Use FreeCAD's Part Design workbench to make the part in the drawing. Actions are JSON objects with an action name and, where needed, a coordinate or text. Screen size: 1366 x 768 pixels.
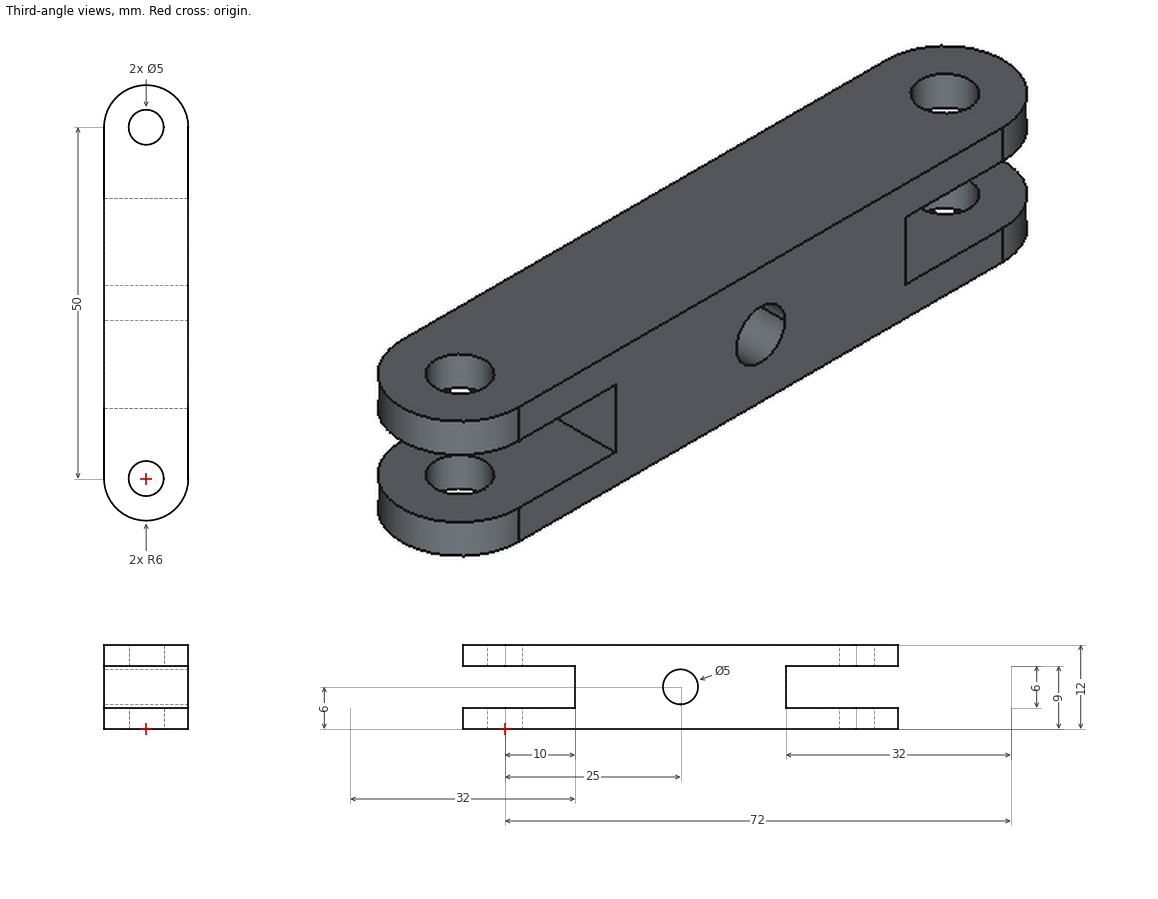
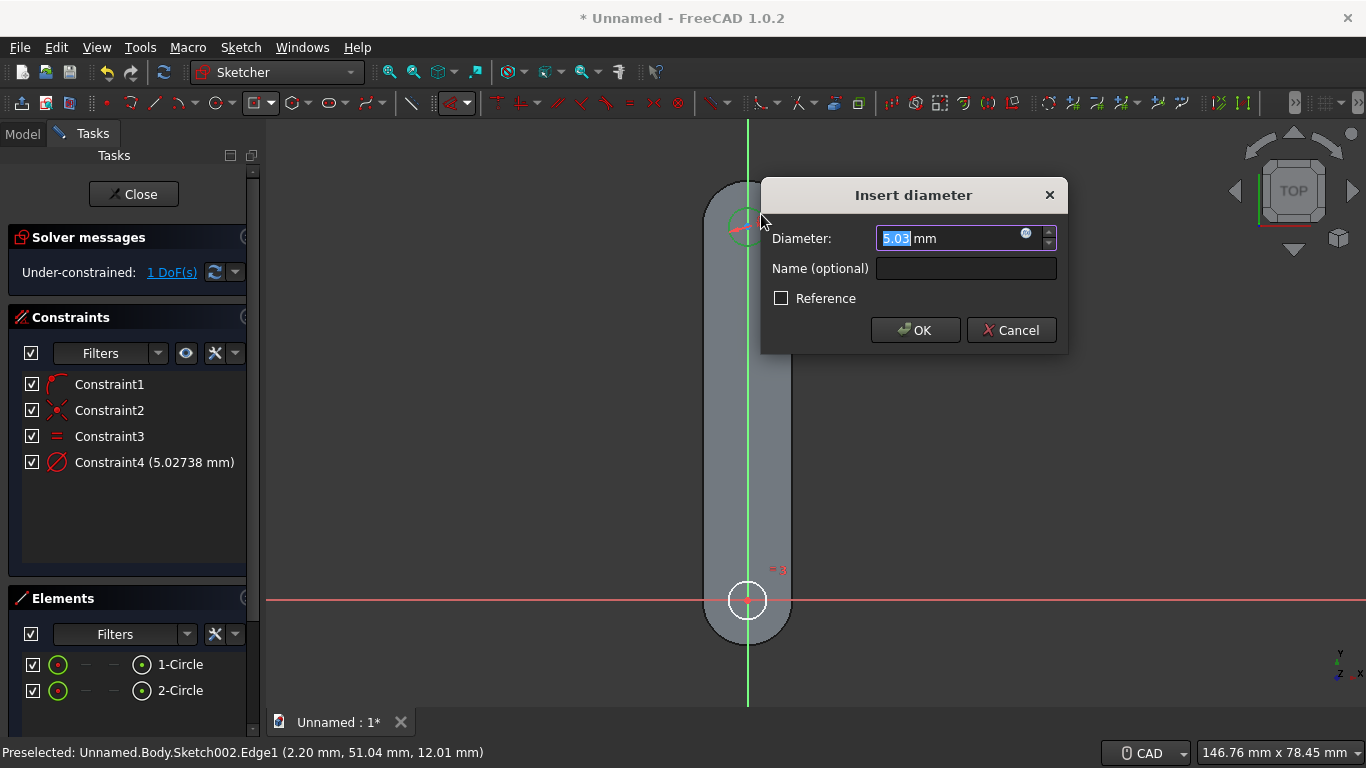
{"action": "type", "text": "5"}
{"action": "key", "text": "Return"}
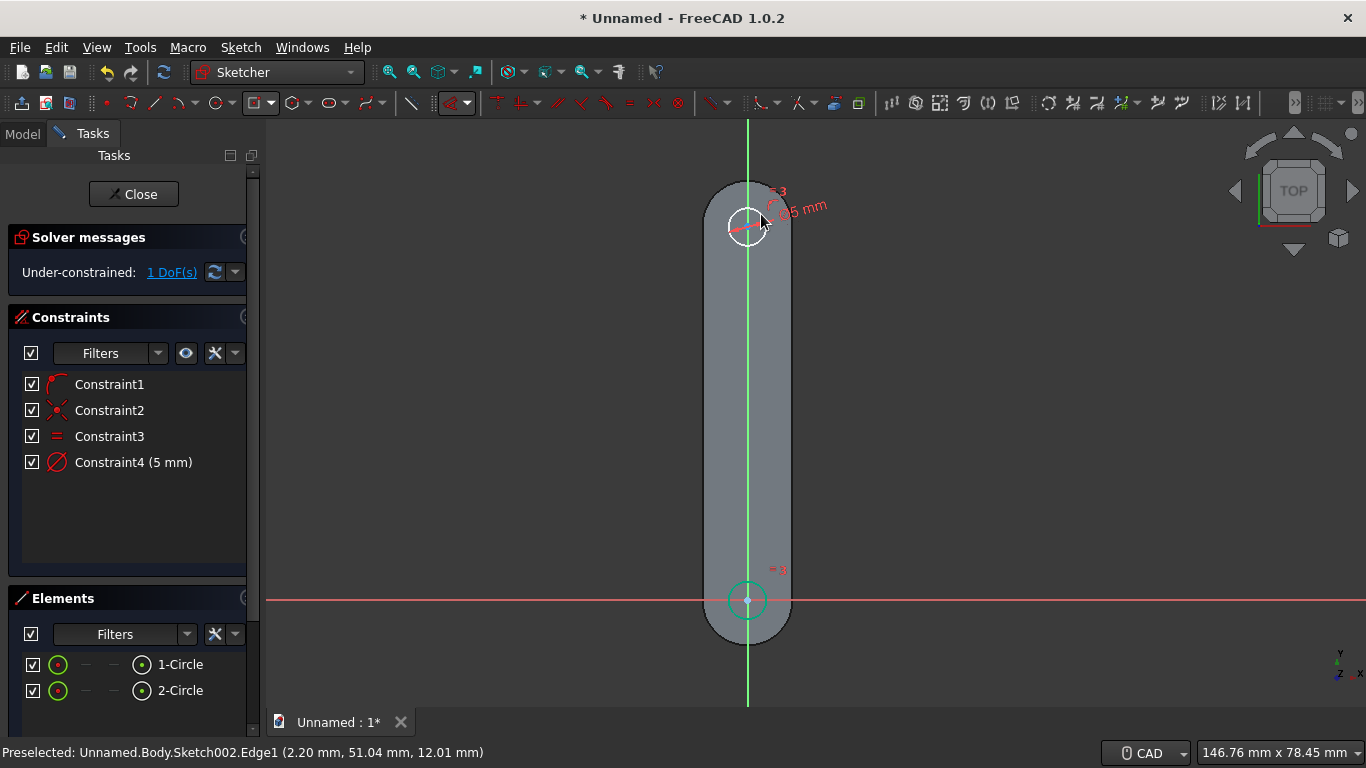
{"action": "left_click", "coordinate": [748, 227]}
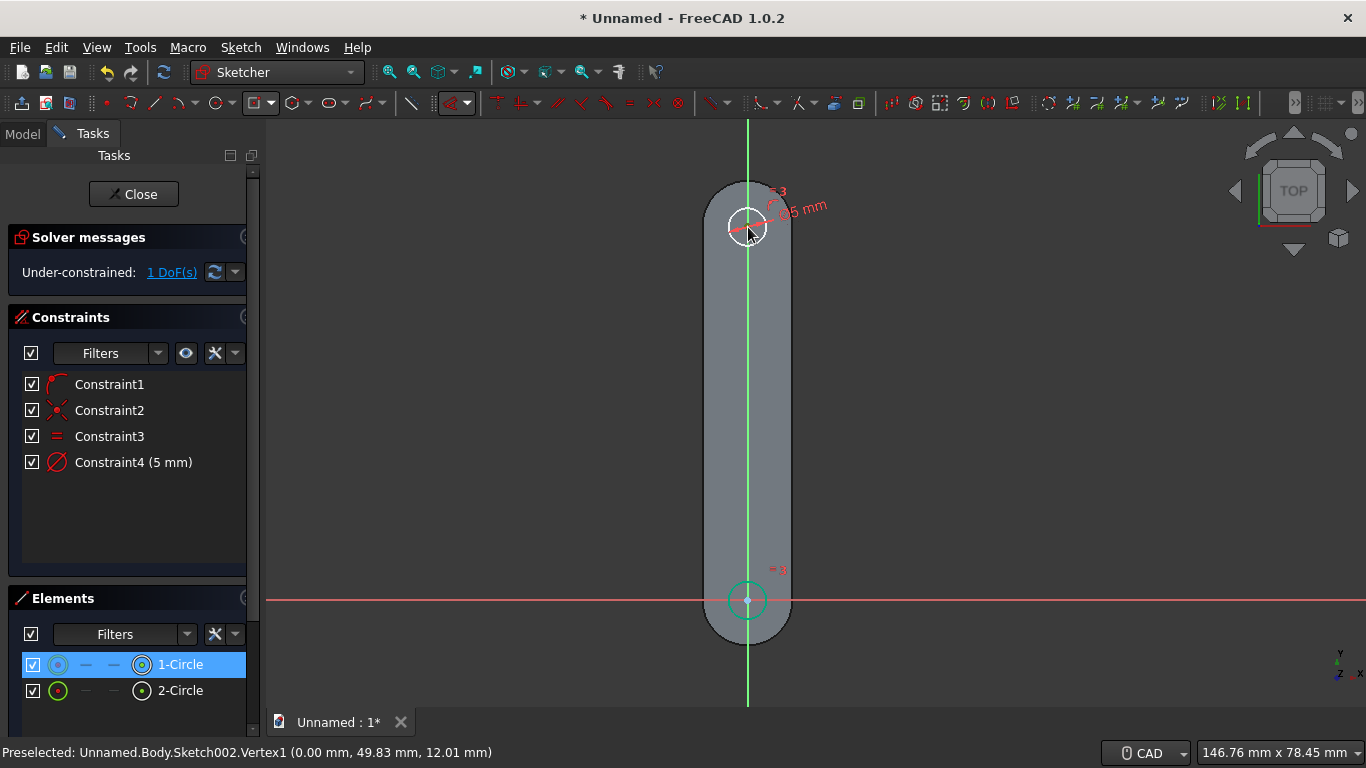
{"action": "left_click", "coordinate": [470, 104]}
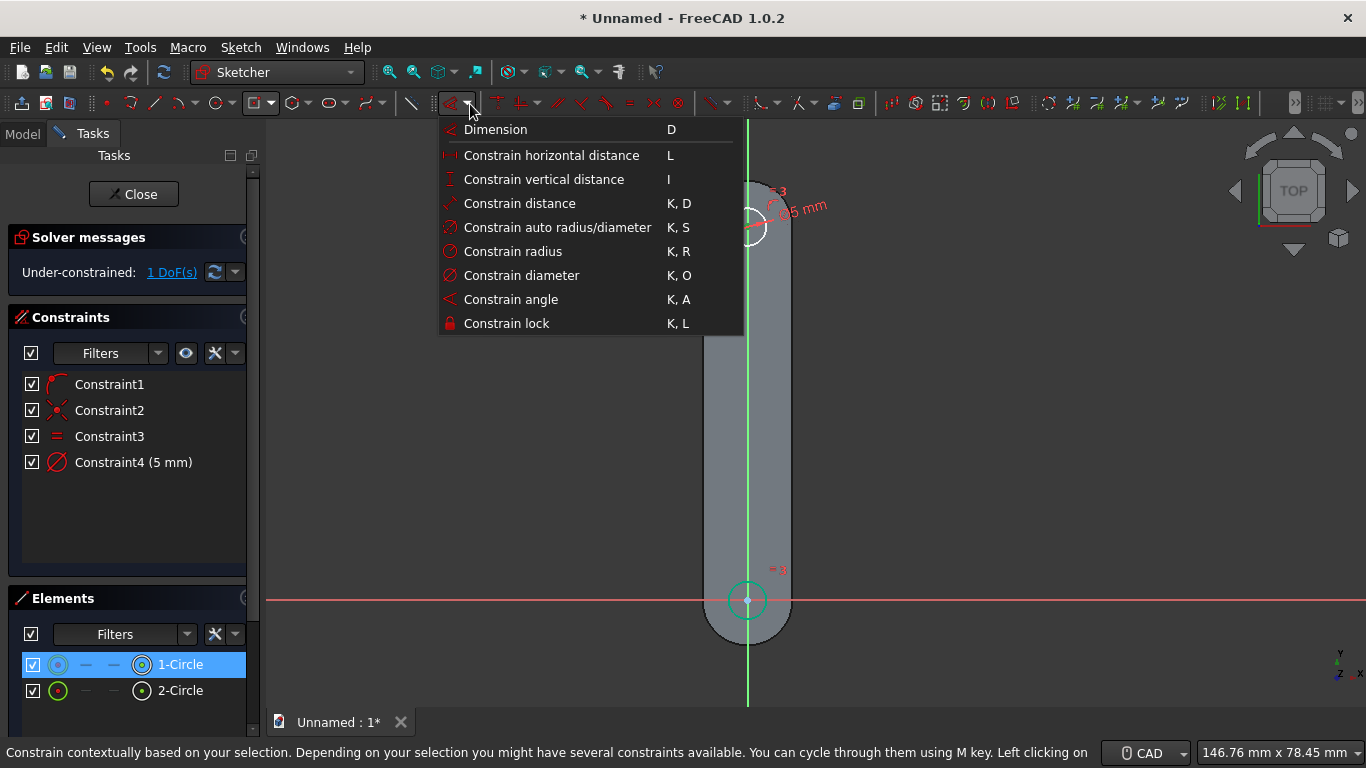
{"action": "left_click", "coordinate": [591, 179]}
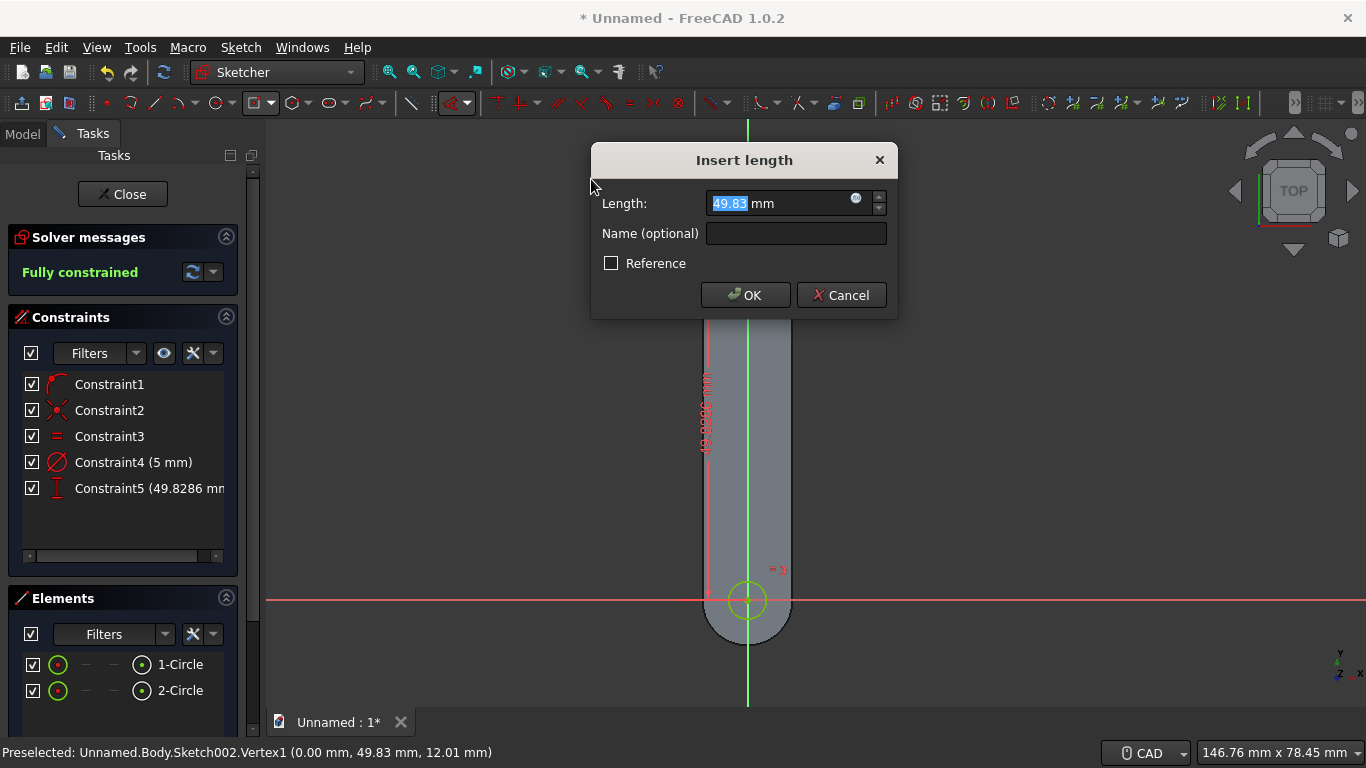
{"action": "type", "text": "50"}
{"action": "key", "text": "Return"}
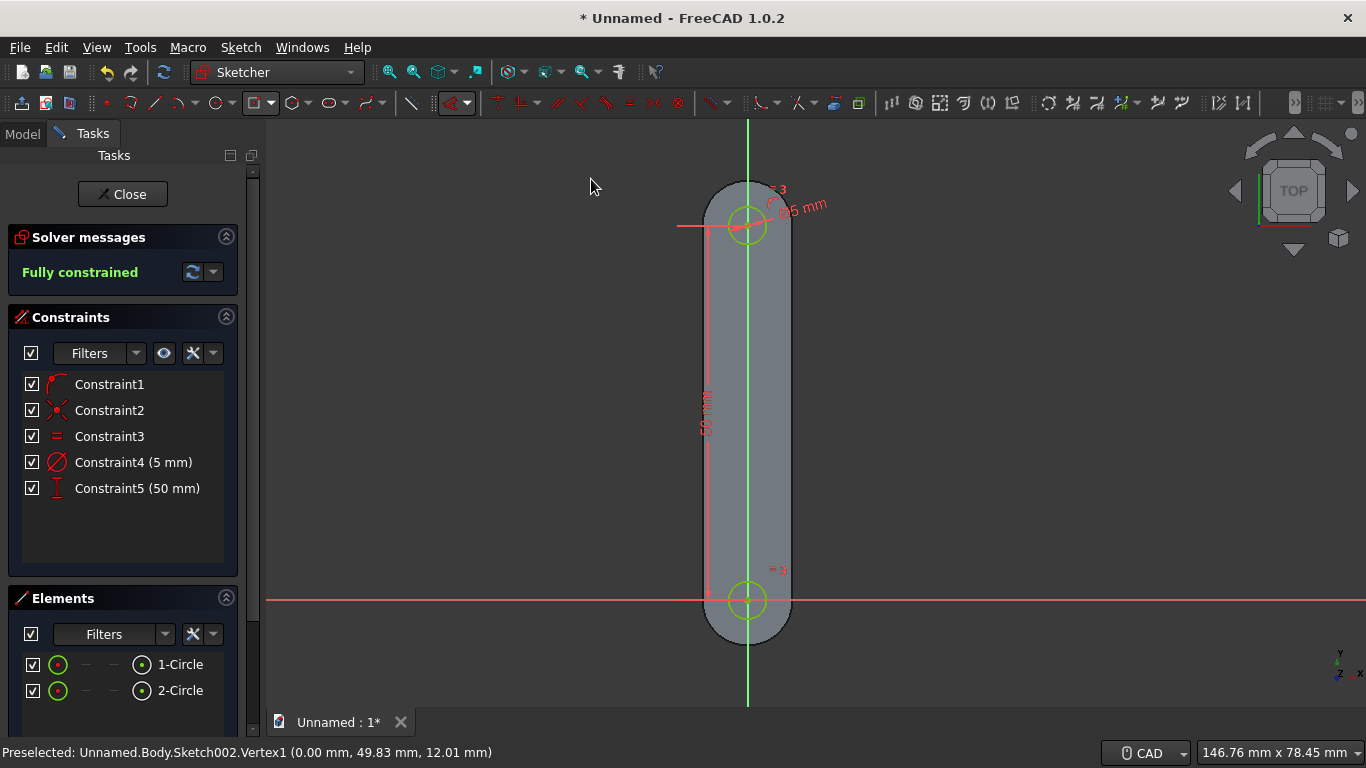
{"action": "left_click", "coordinate": [123, 194]}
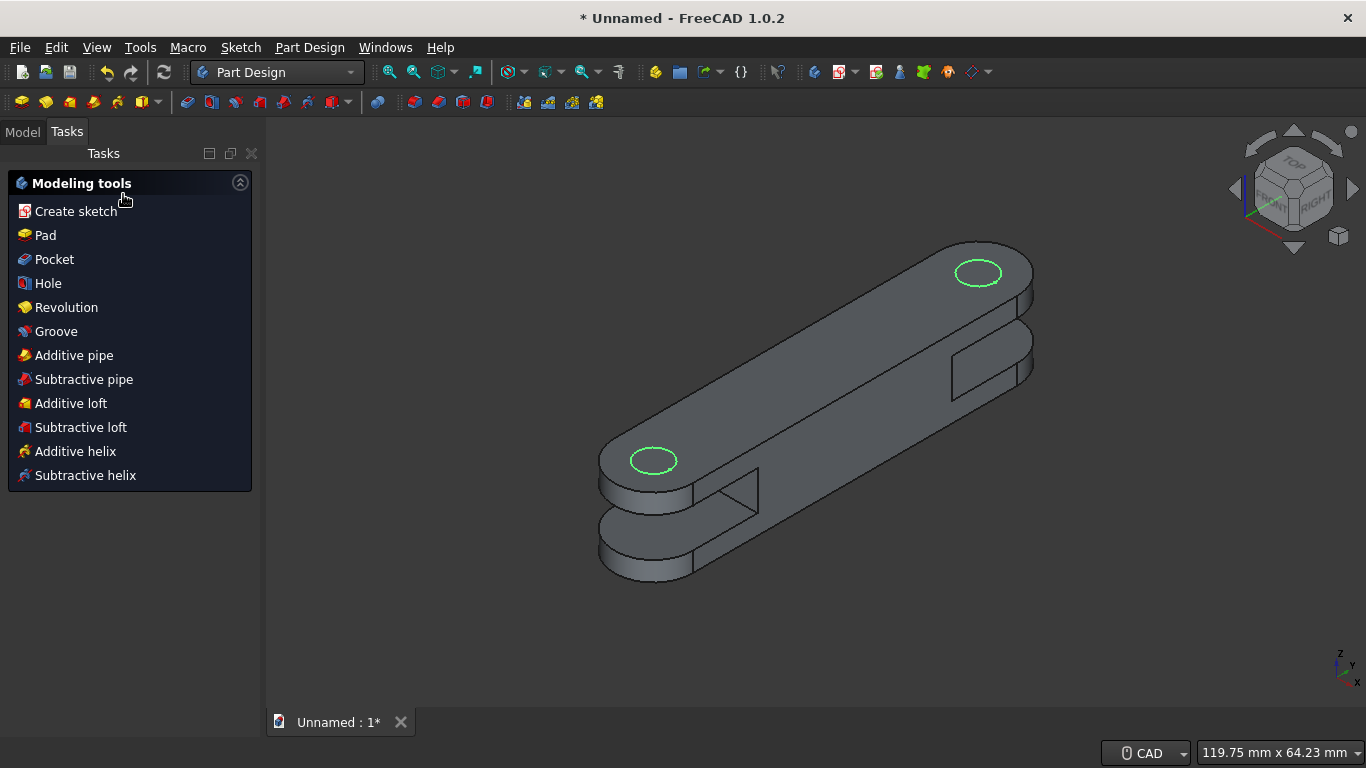
{"action": "left_click", "coordinate": [188, 102]}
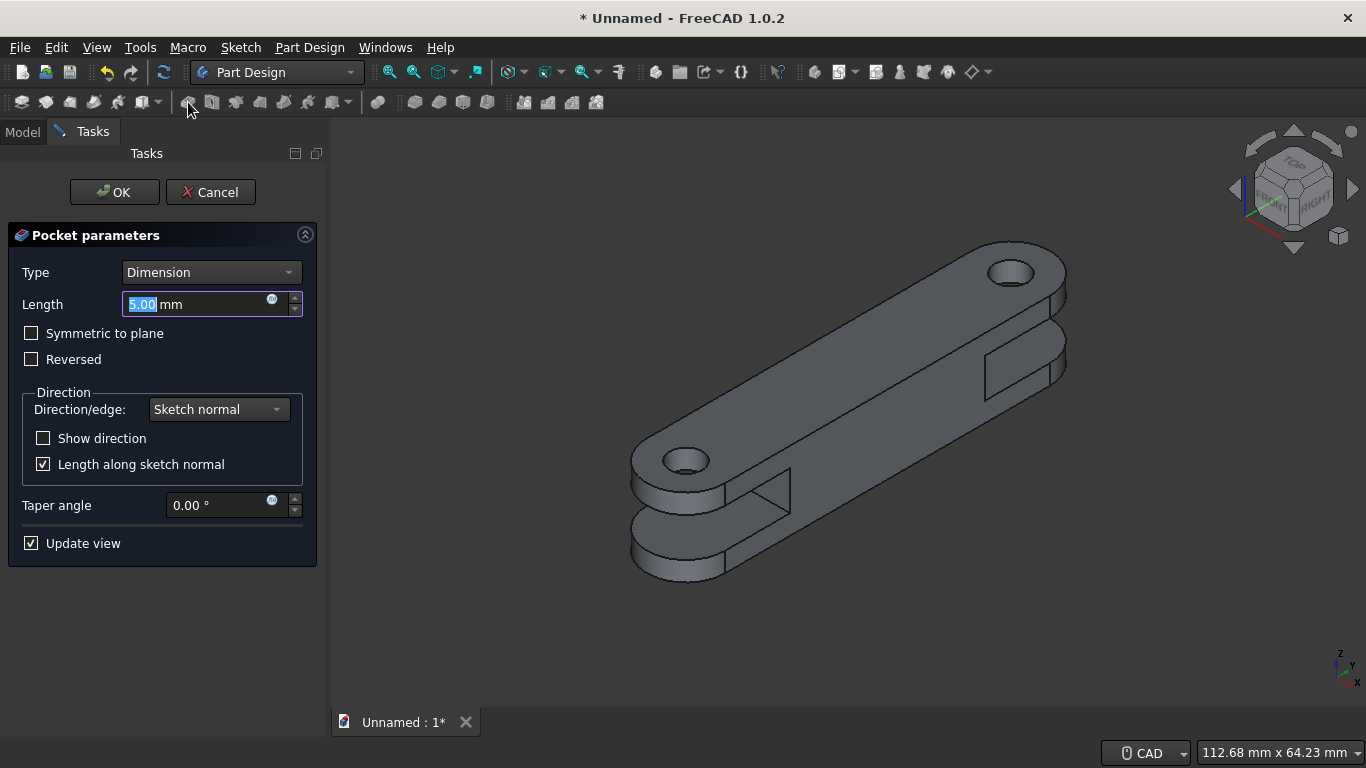
{"action": "left_click", "coordinate": [212, 272]}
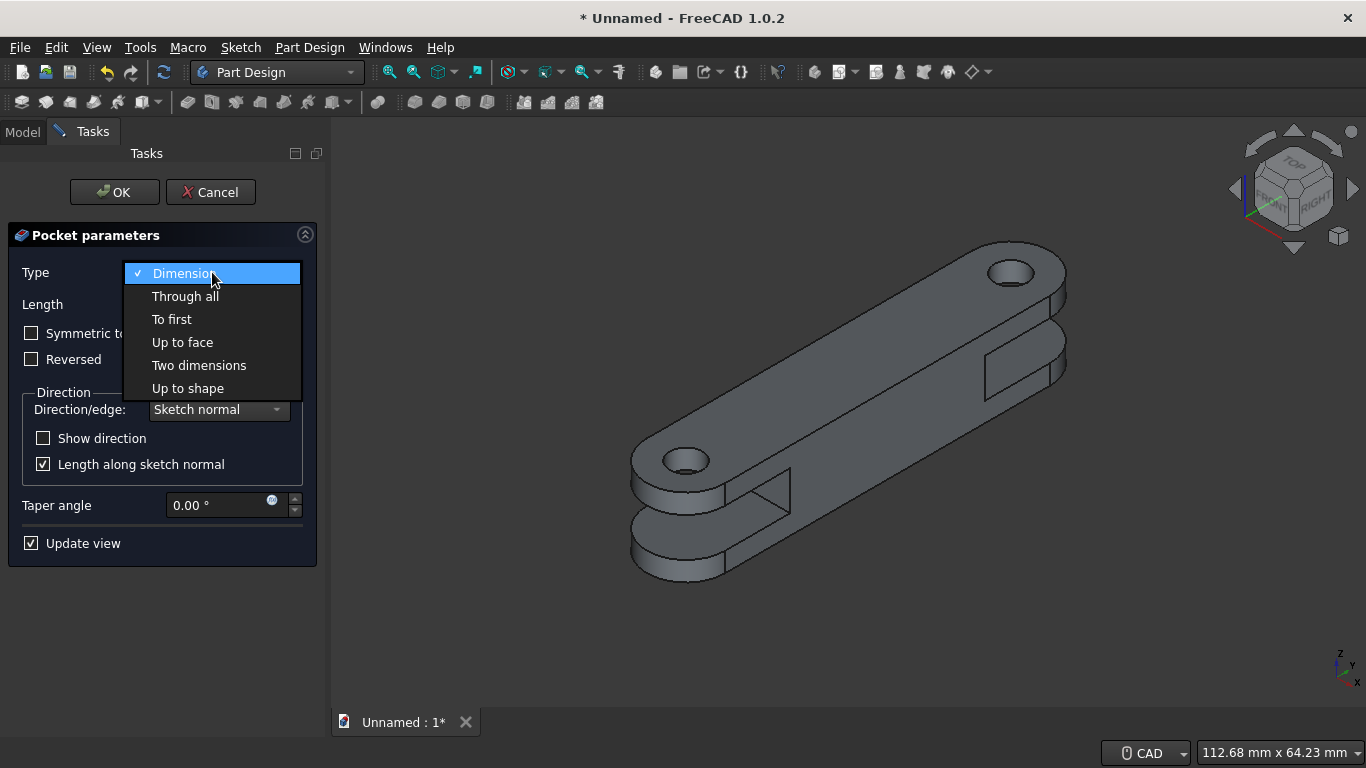
{"action": "left_click", "coordinate": [212, 296]}